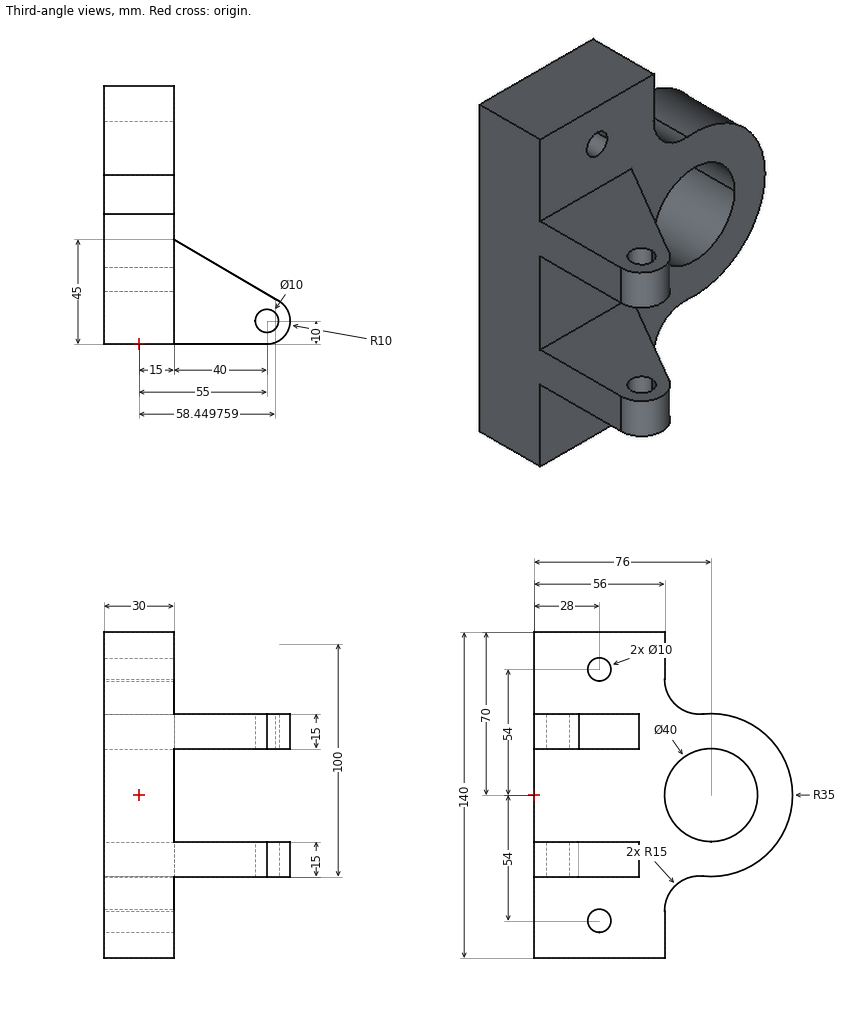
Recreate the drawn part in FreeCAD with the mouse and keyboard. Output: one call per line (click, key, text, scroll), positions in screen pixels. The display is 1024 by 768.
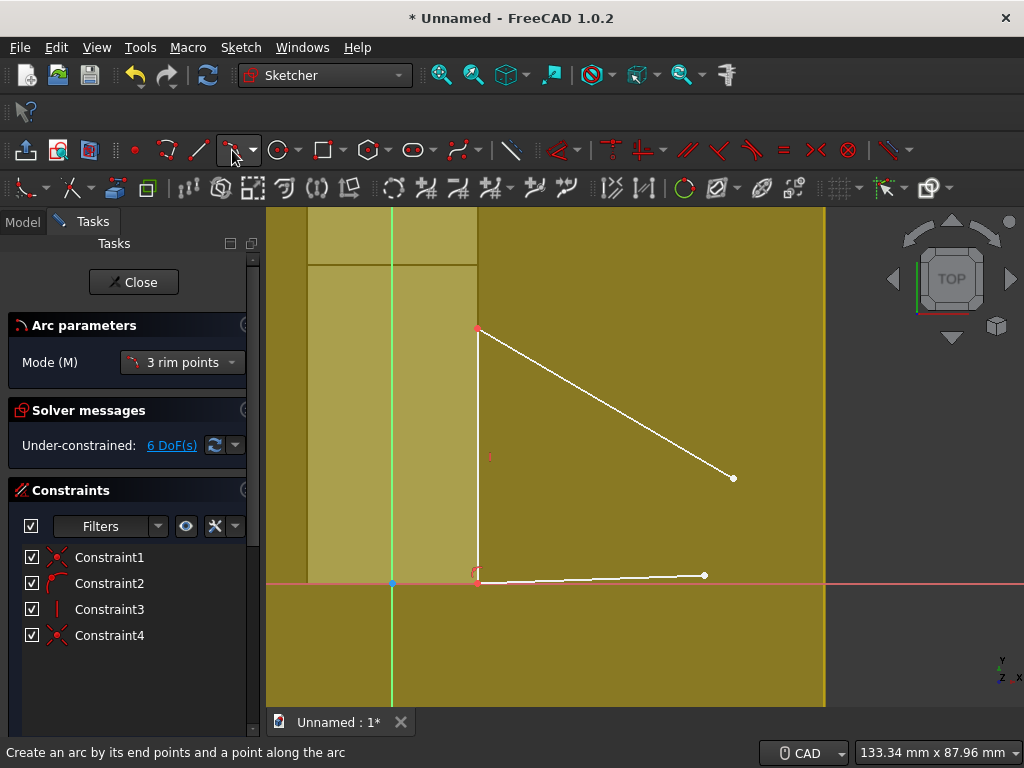
click(705, 576)
click(734, 479)
click(760, 542)
key(Escape)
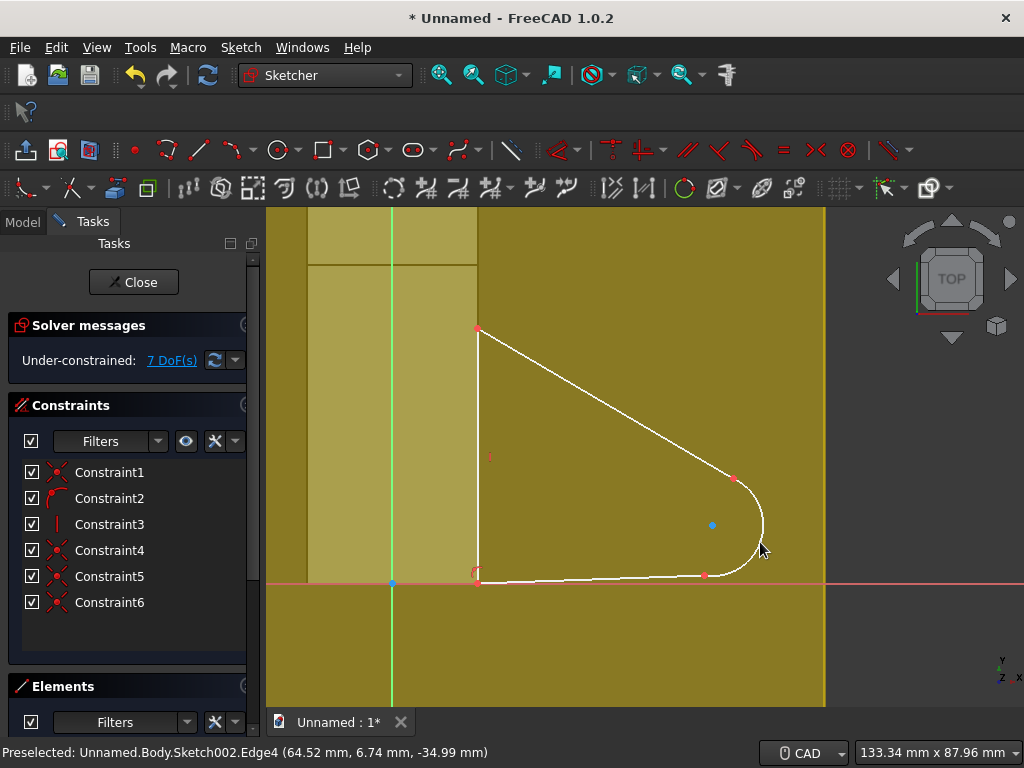
click(657, 434)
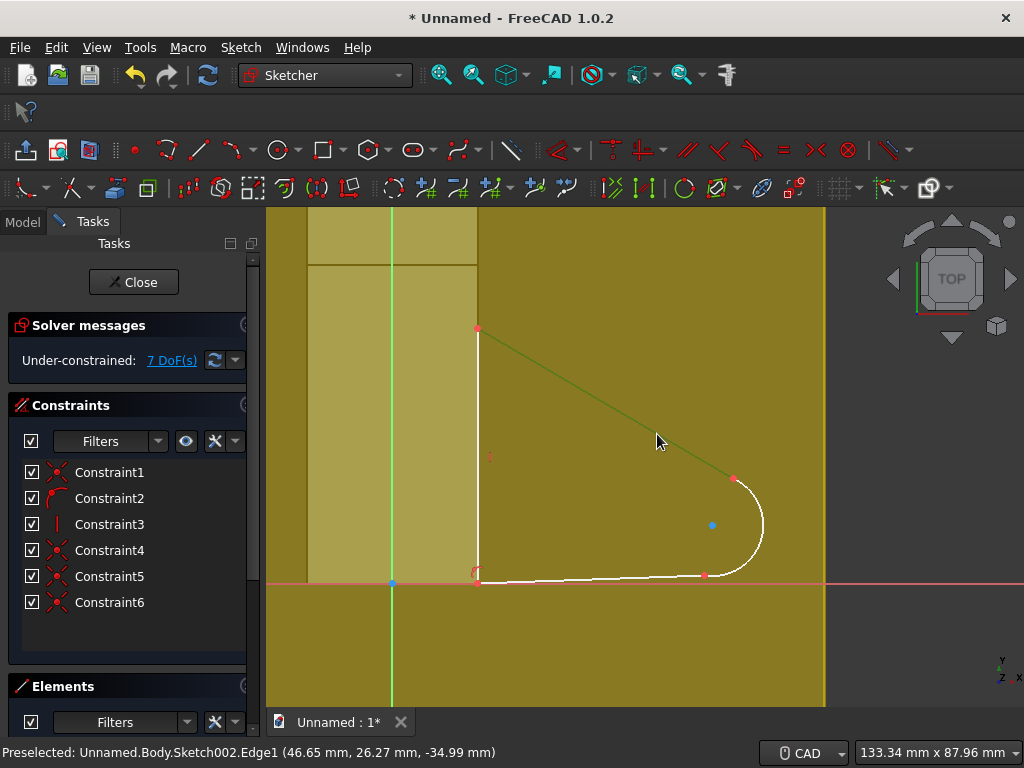
click(745, 564)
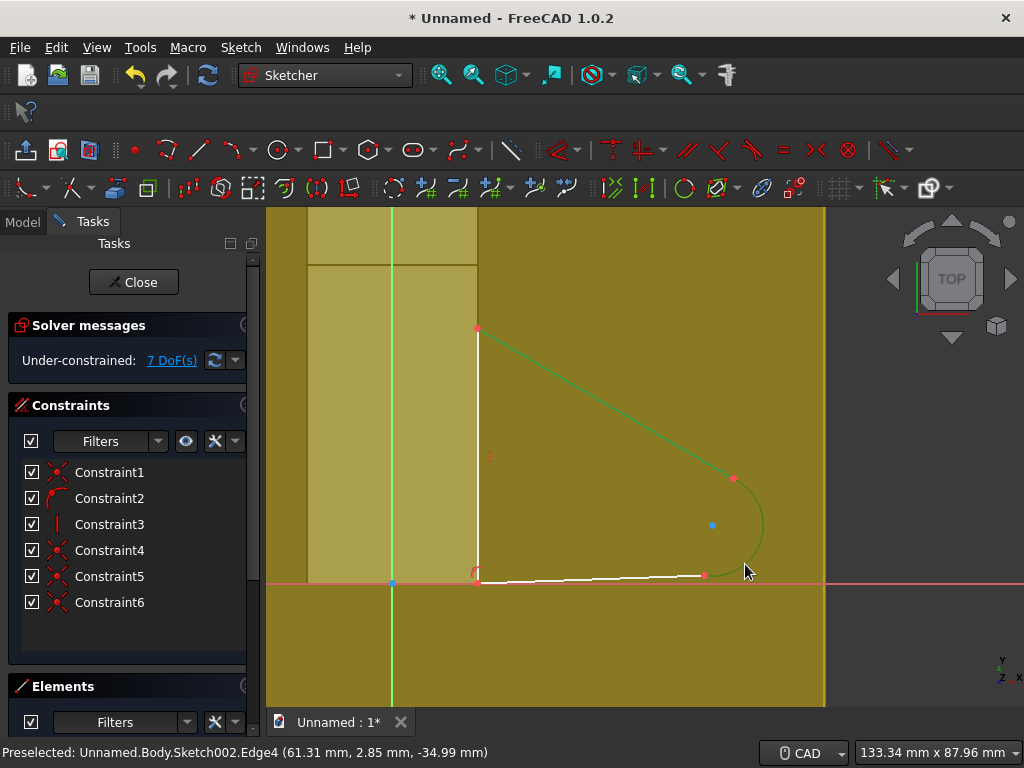
key(t)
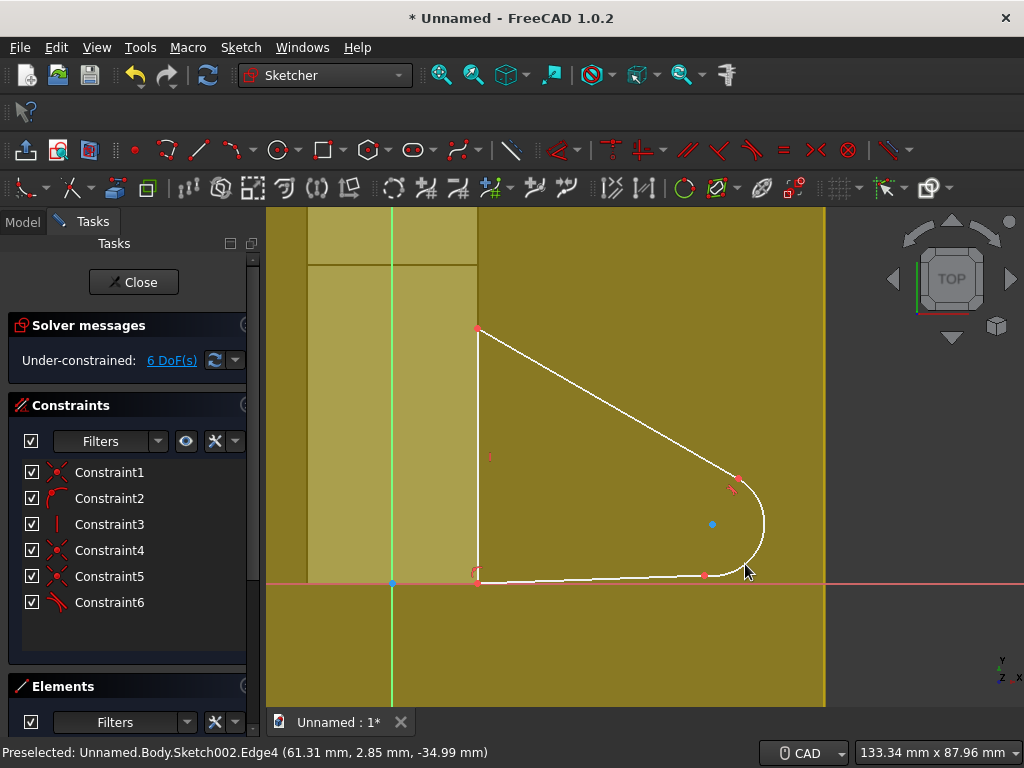
click(546, 581)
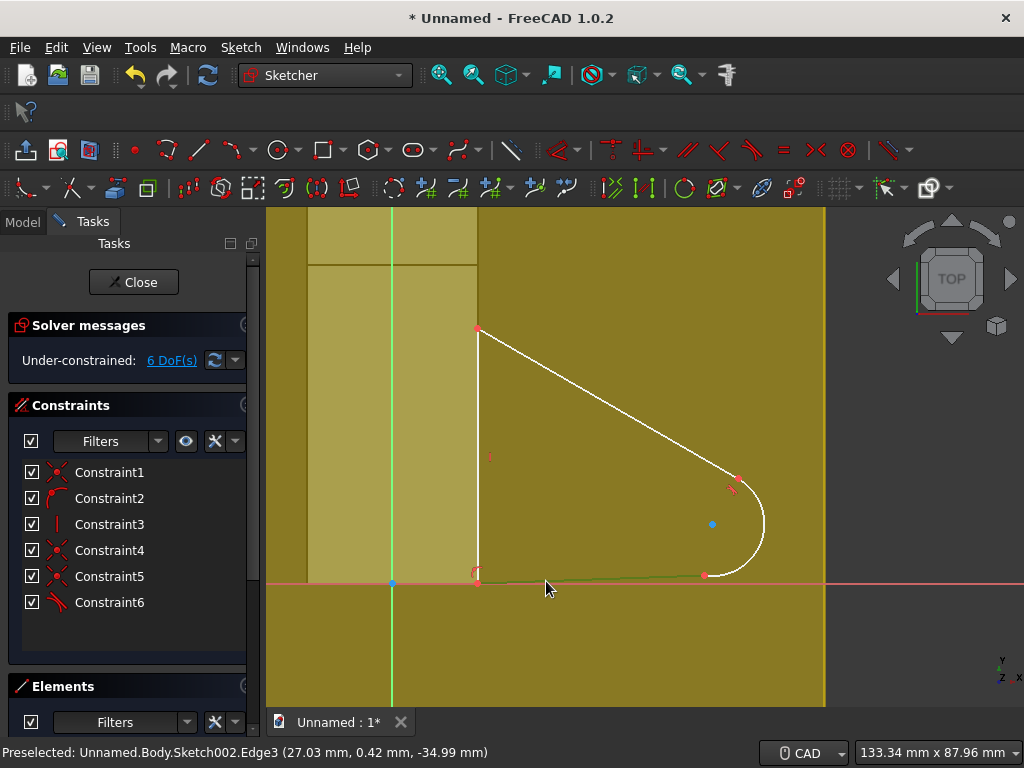
click(745, 564)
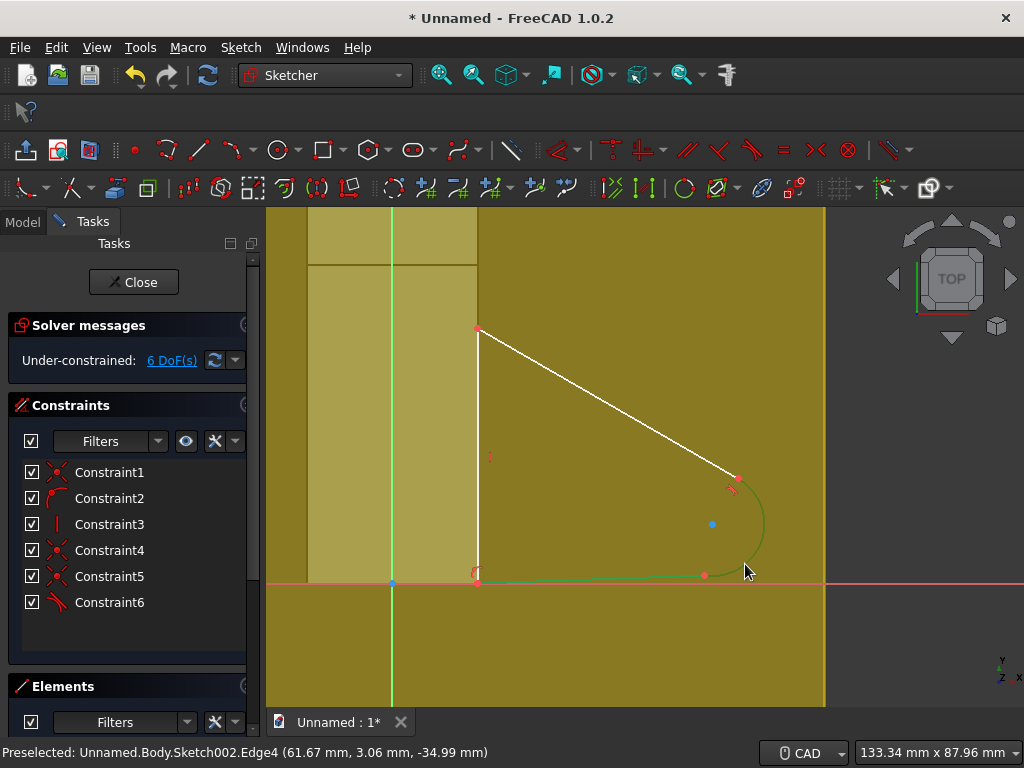
key(t)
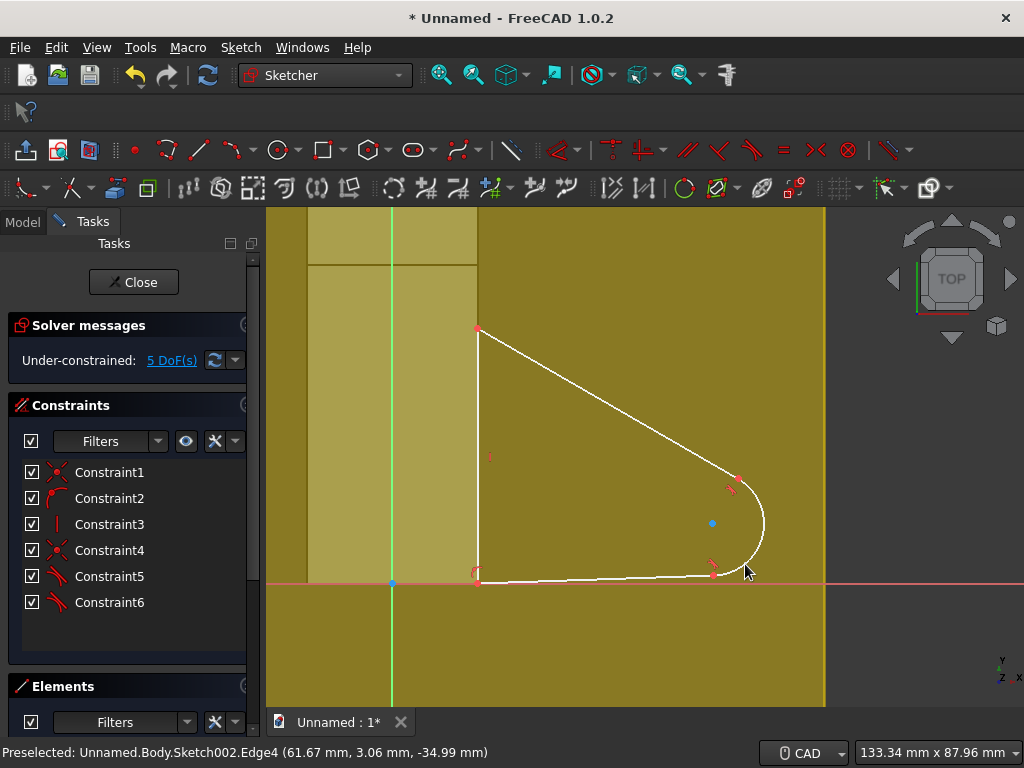
click(549, 581)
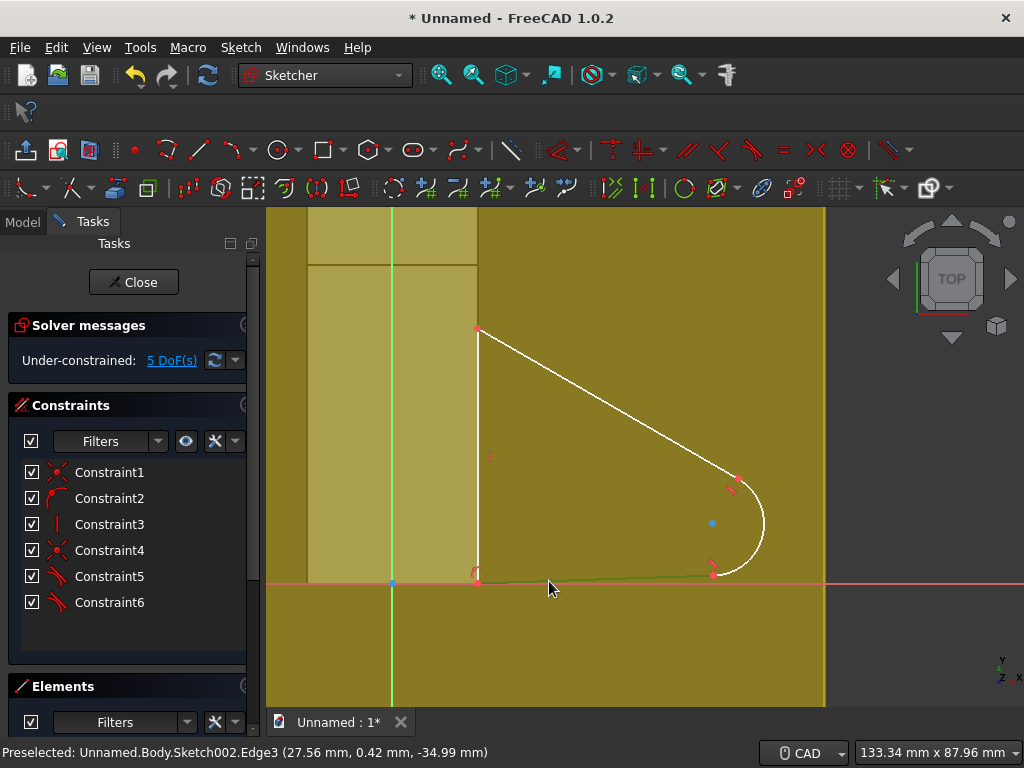
key(h)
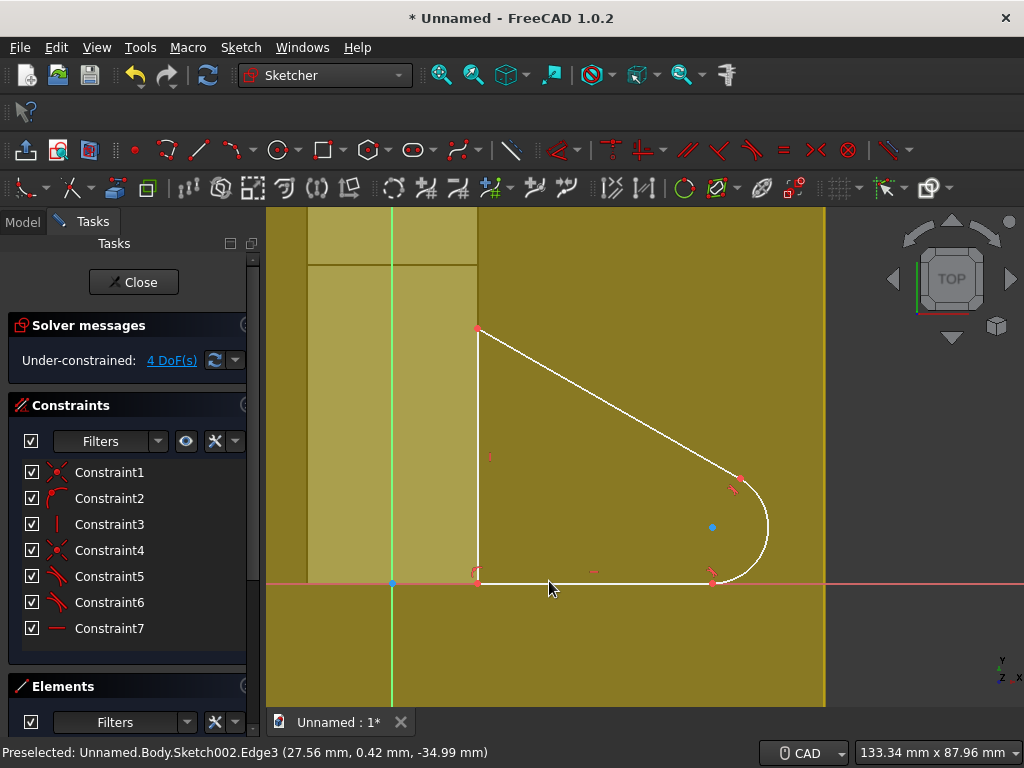
key(d)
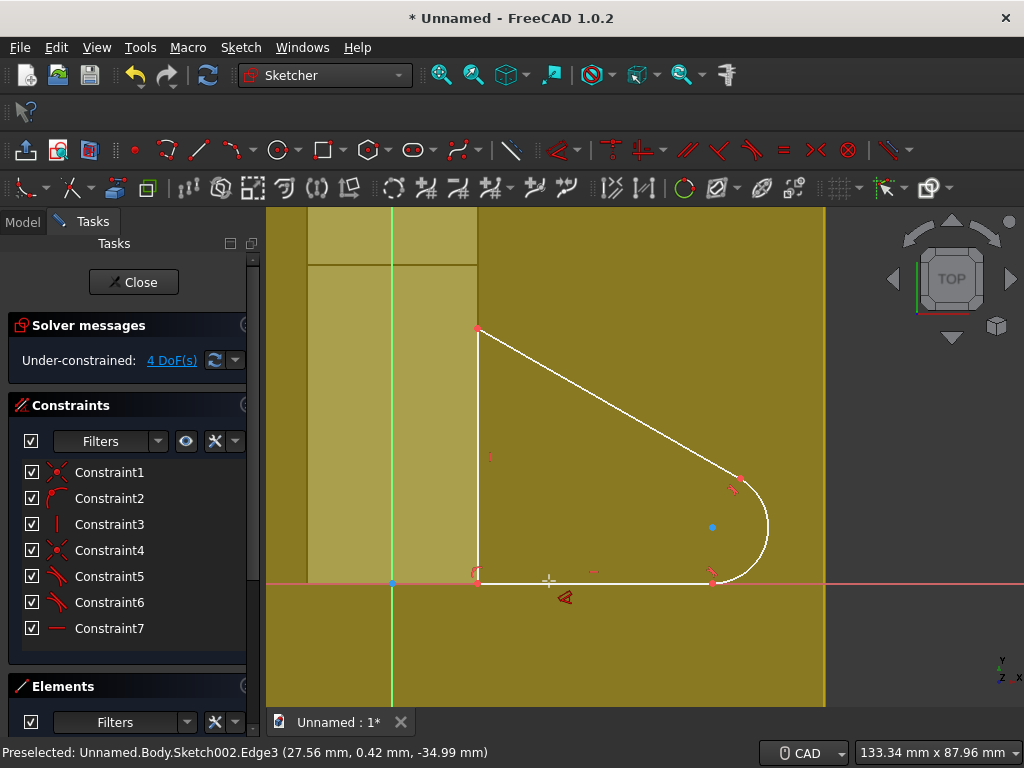
click(752, 567)
click(737, 612)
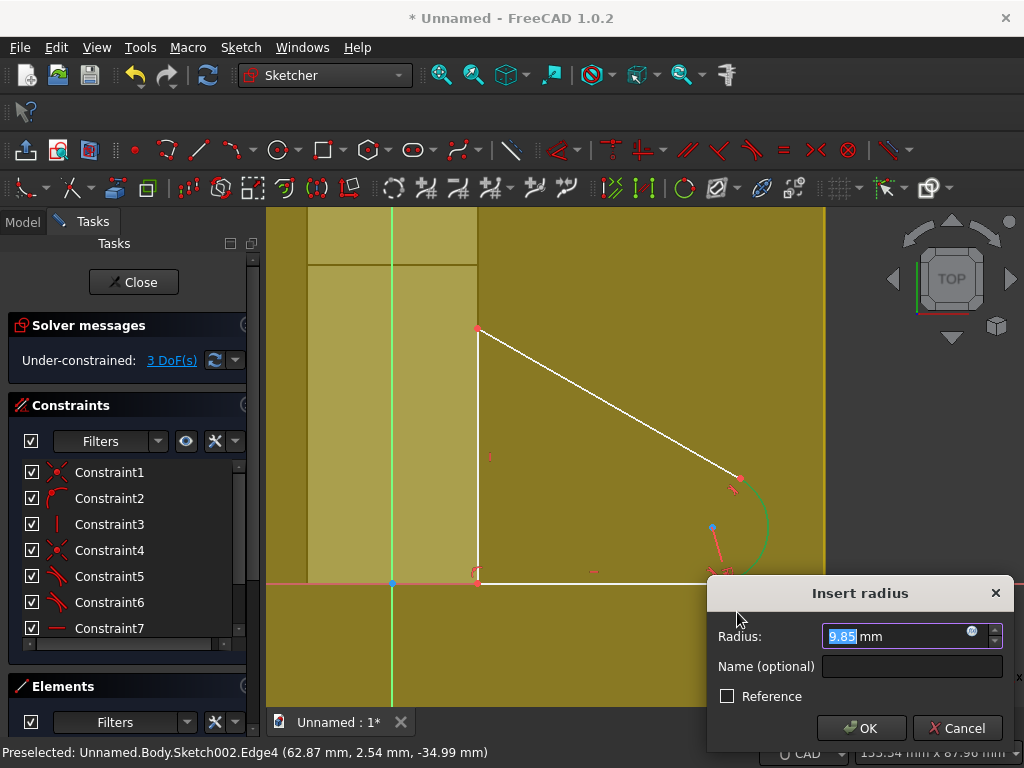
text(10)
key(Return)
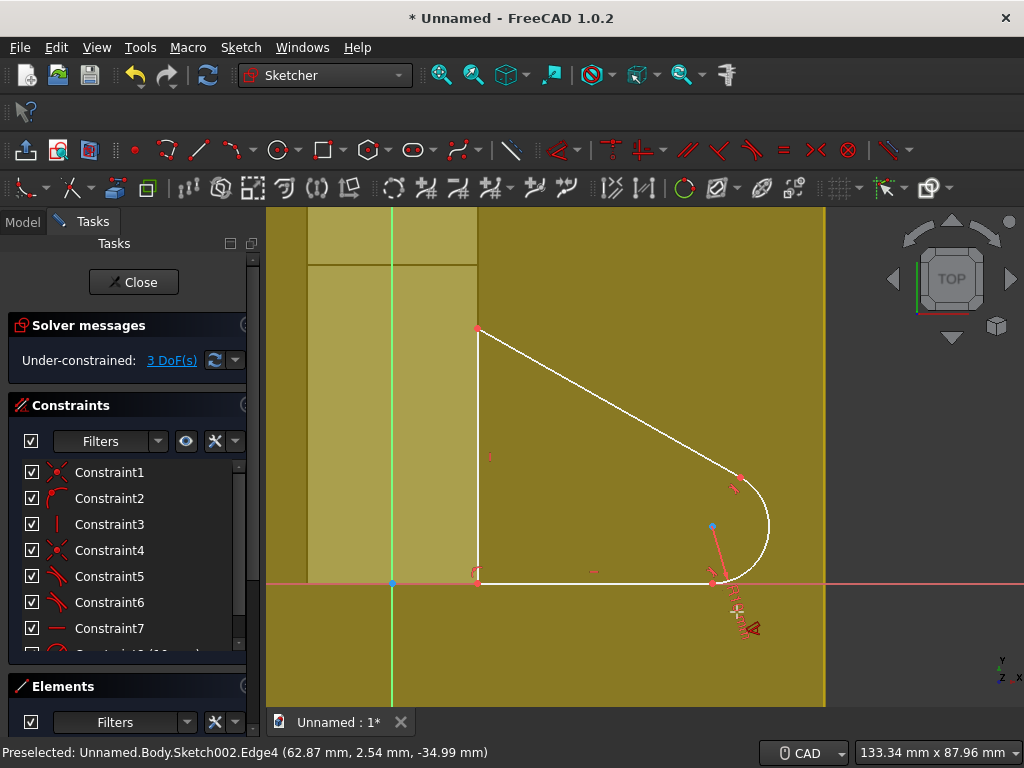
click(478, 405)
click(444, 456)